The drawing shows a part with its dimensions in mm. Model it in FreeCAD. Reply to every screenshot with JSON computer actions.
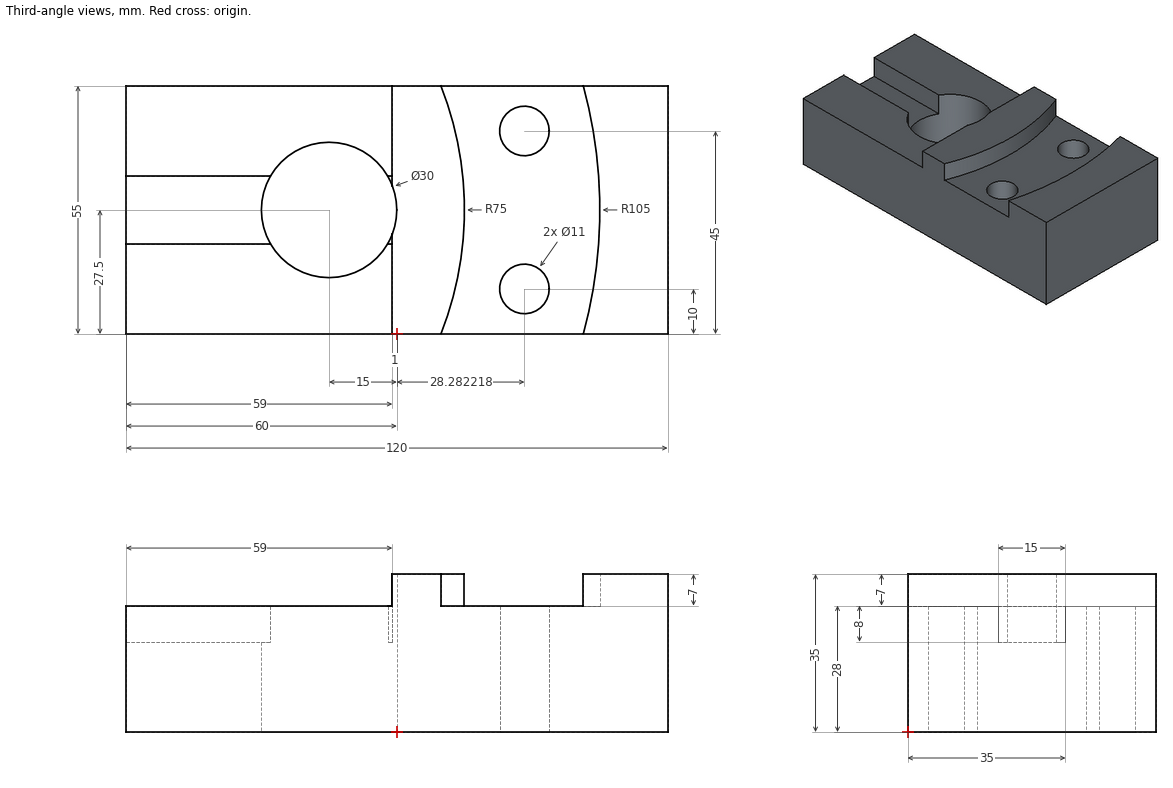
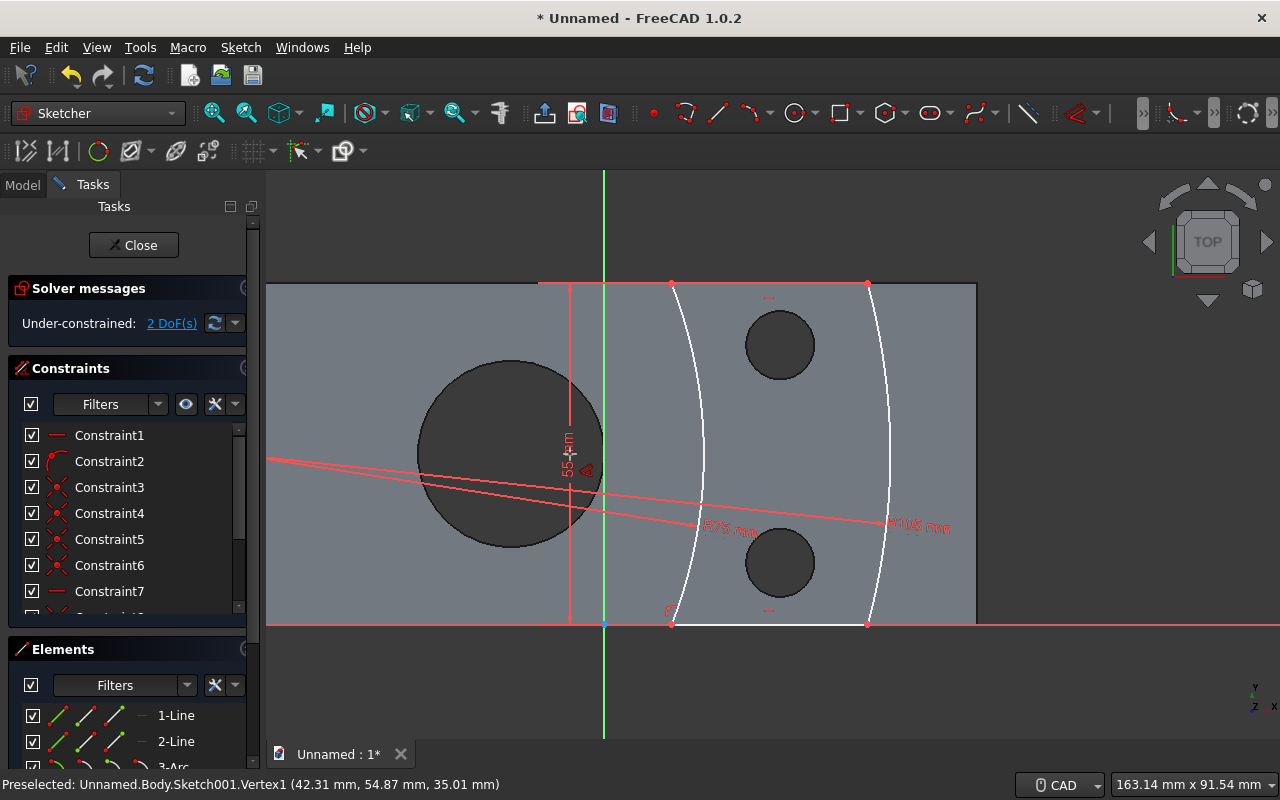
{"action": "scroll", "coordinate": [1115, 457], "scroll_direction": "down", "scroll_amount": 1}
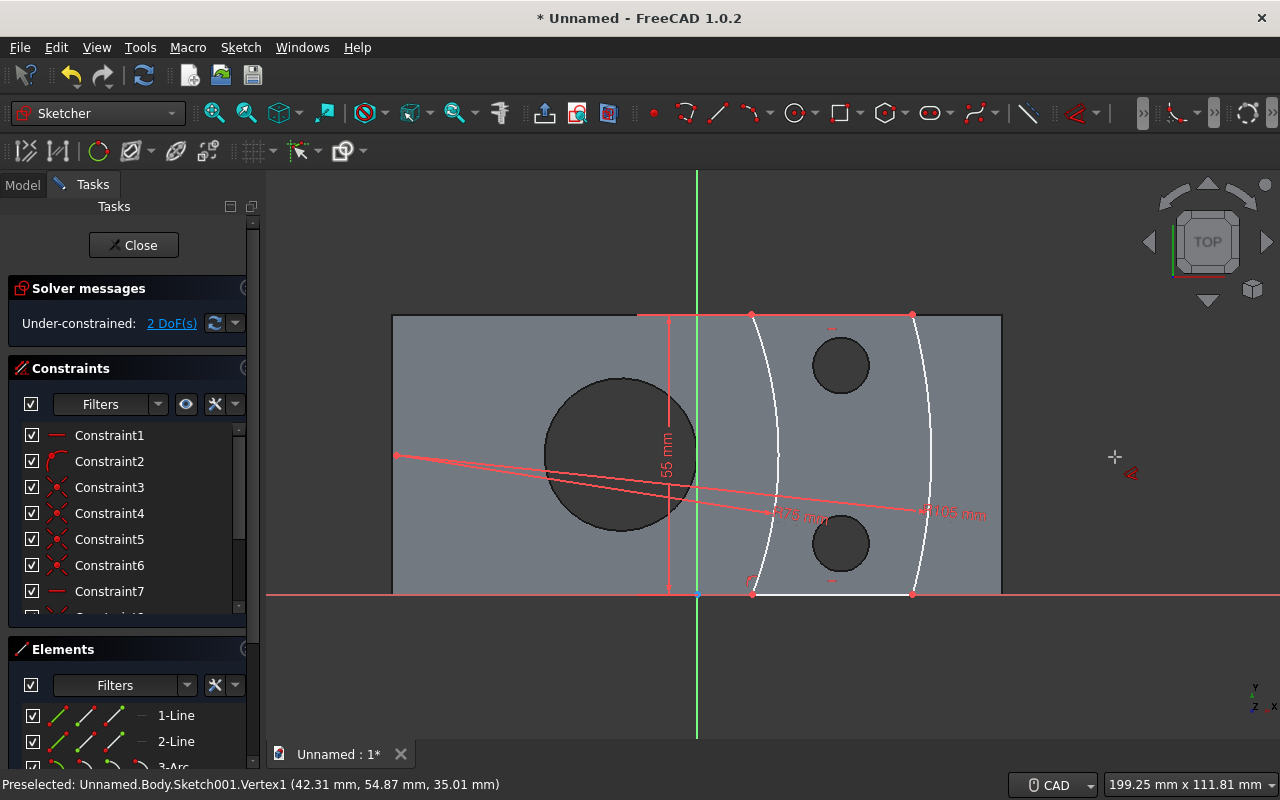
{"action": "left_click", "coordinate": [397, 455]}
{"action": "left_click", "coordinate": [547, 629]}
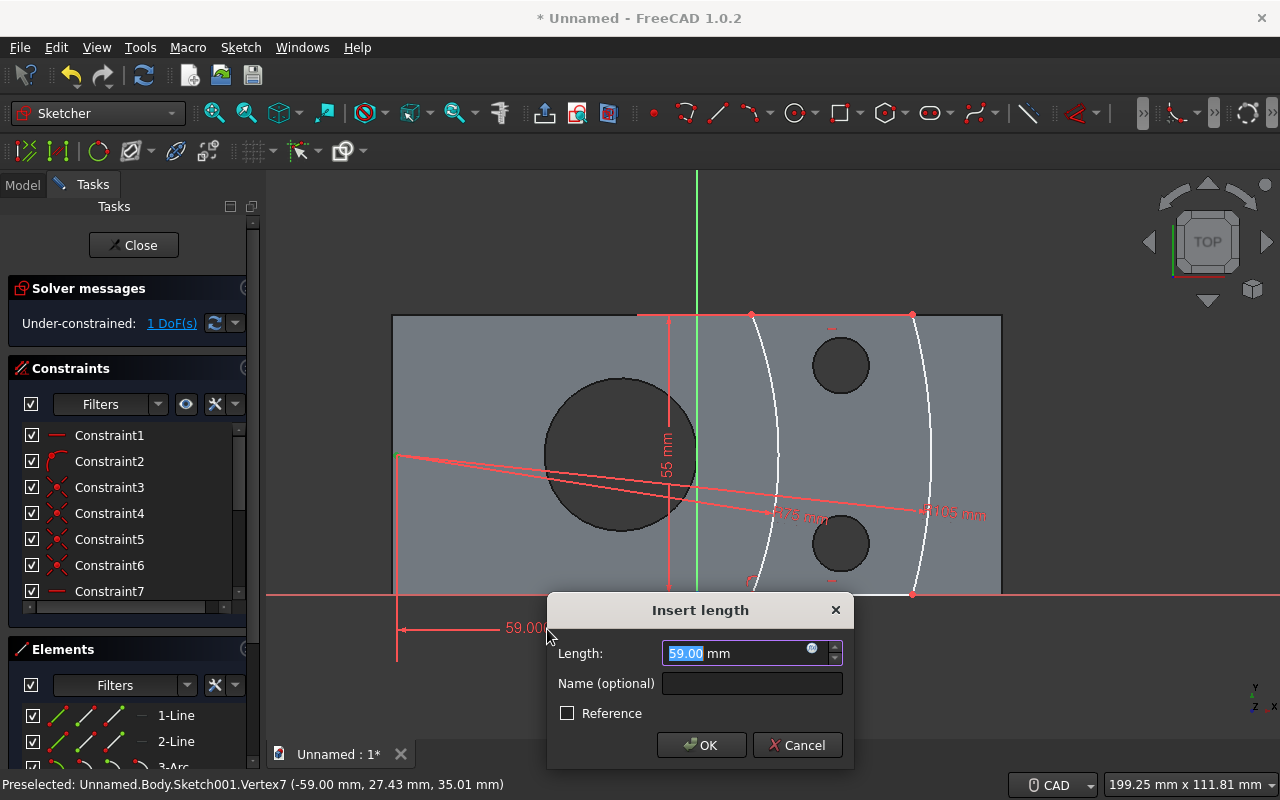
{"action": "type", "text": "60"}
{"action": "key", "text": "Return"}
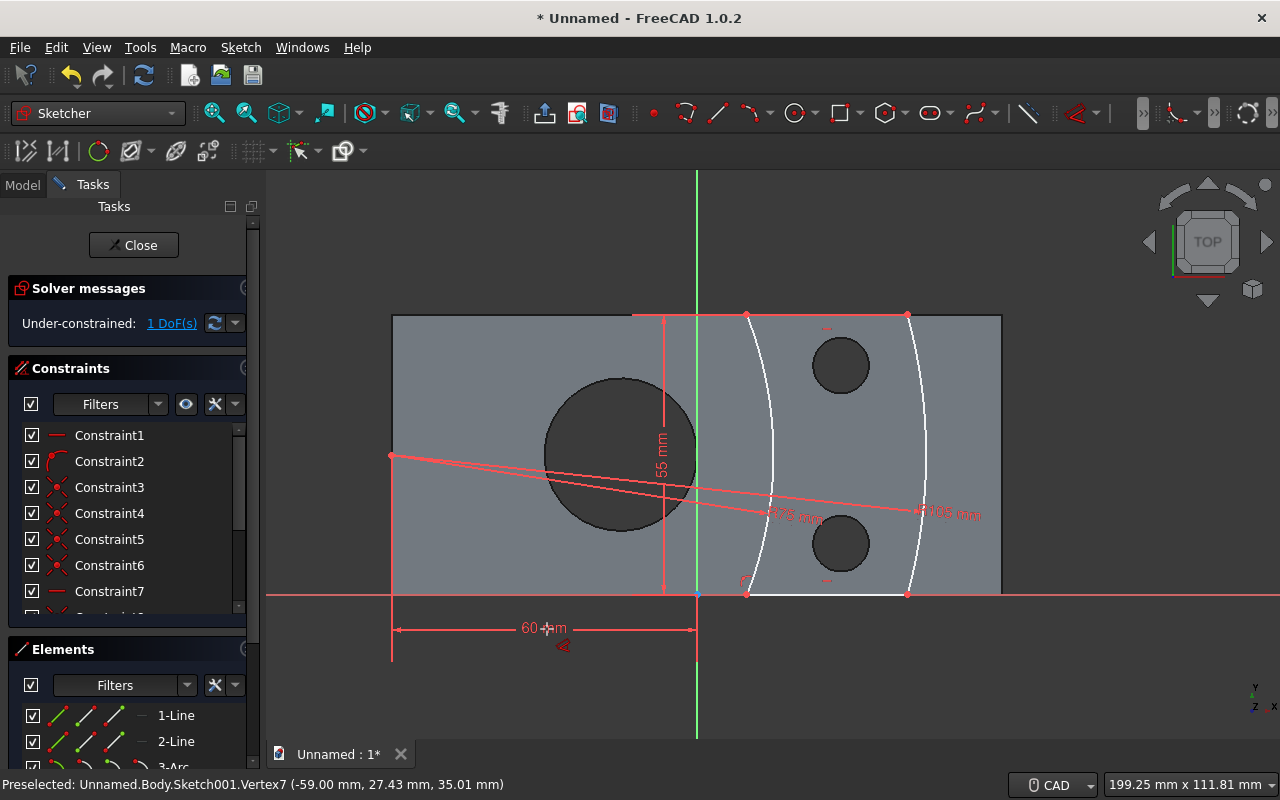
{"action": "left_click", "coordinate": [392, 455]}
{"action": "left_click", "coordinate": [358, 525]}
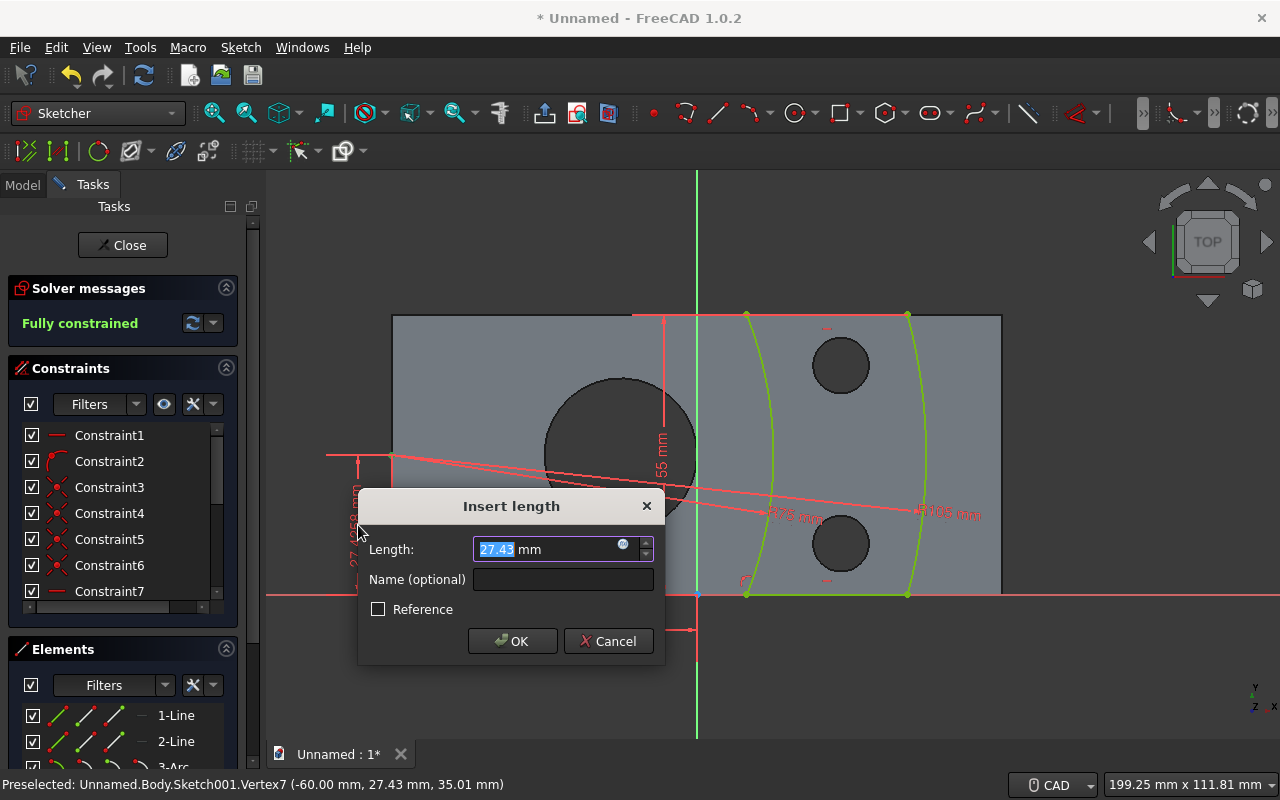
{"action": "type", "text": "27.5"}
{"action": "key", "text": "Return"}
{"action": "key", "text": "Escape"}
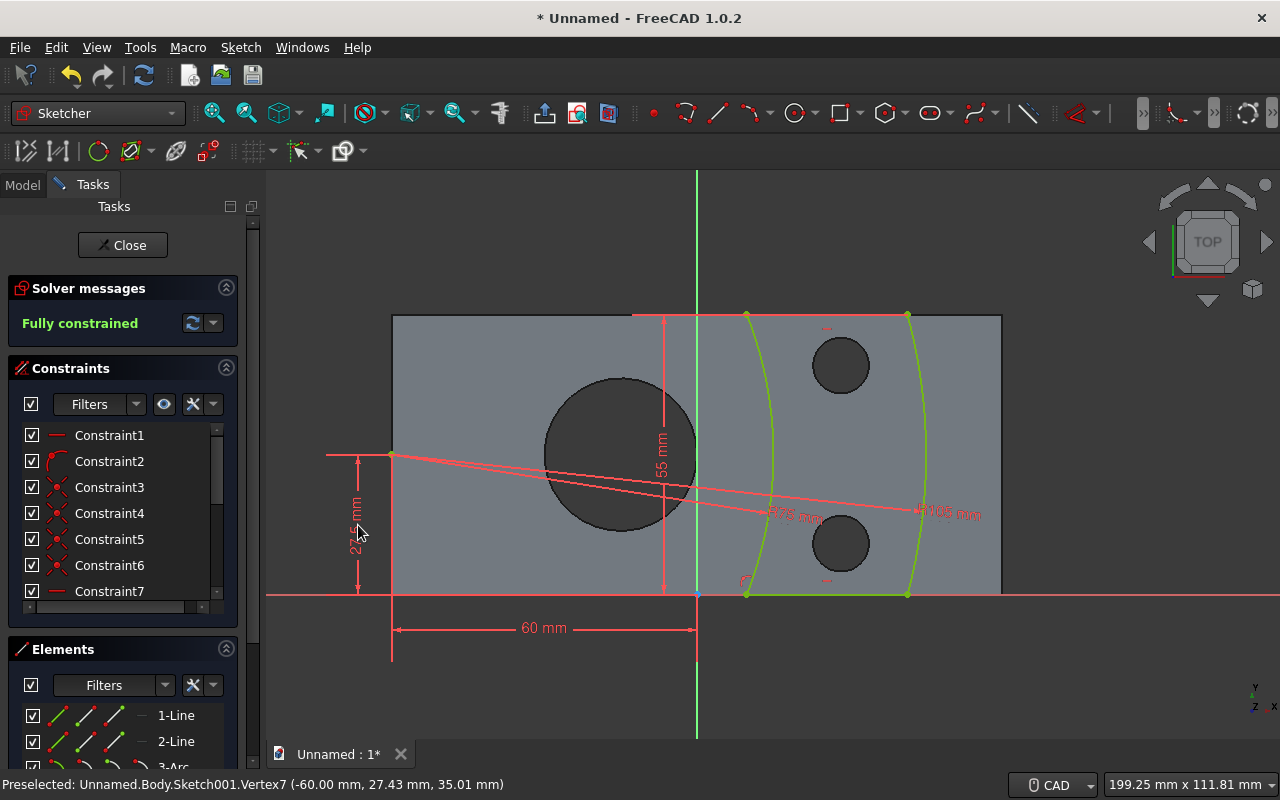
{"action": "left_click", "coordinate": [123, 245]}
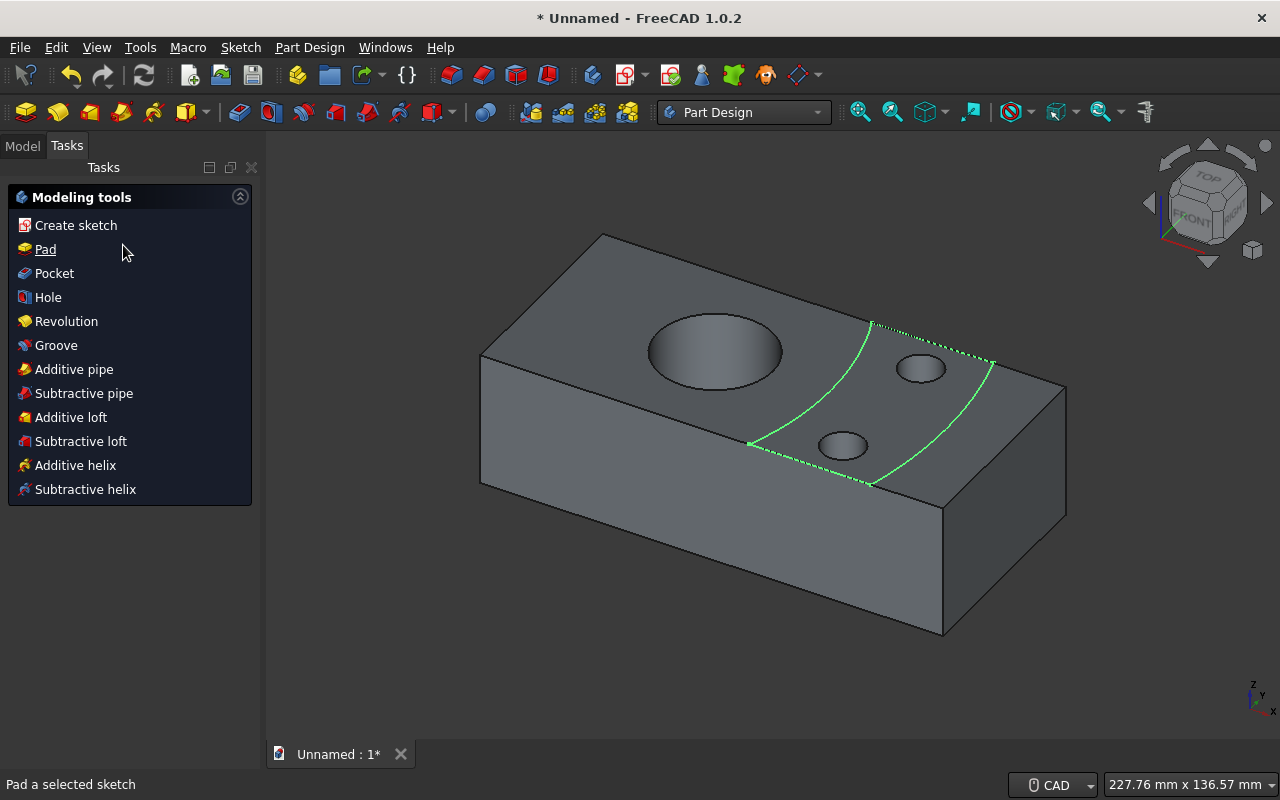
{"action": "left_click", "coordinate": [240, 112]}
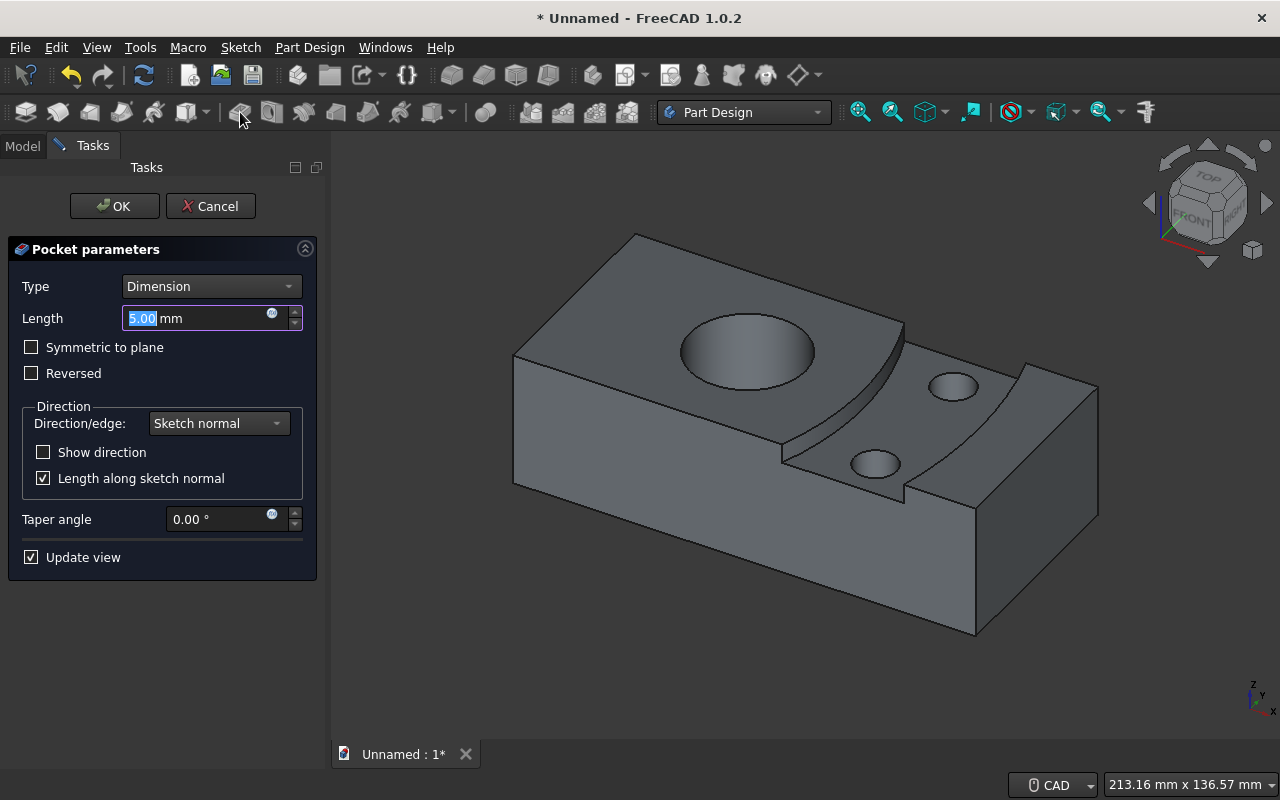
{"action": "type", "text": "7"}
{"action": "key", "text": "Tab"}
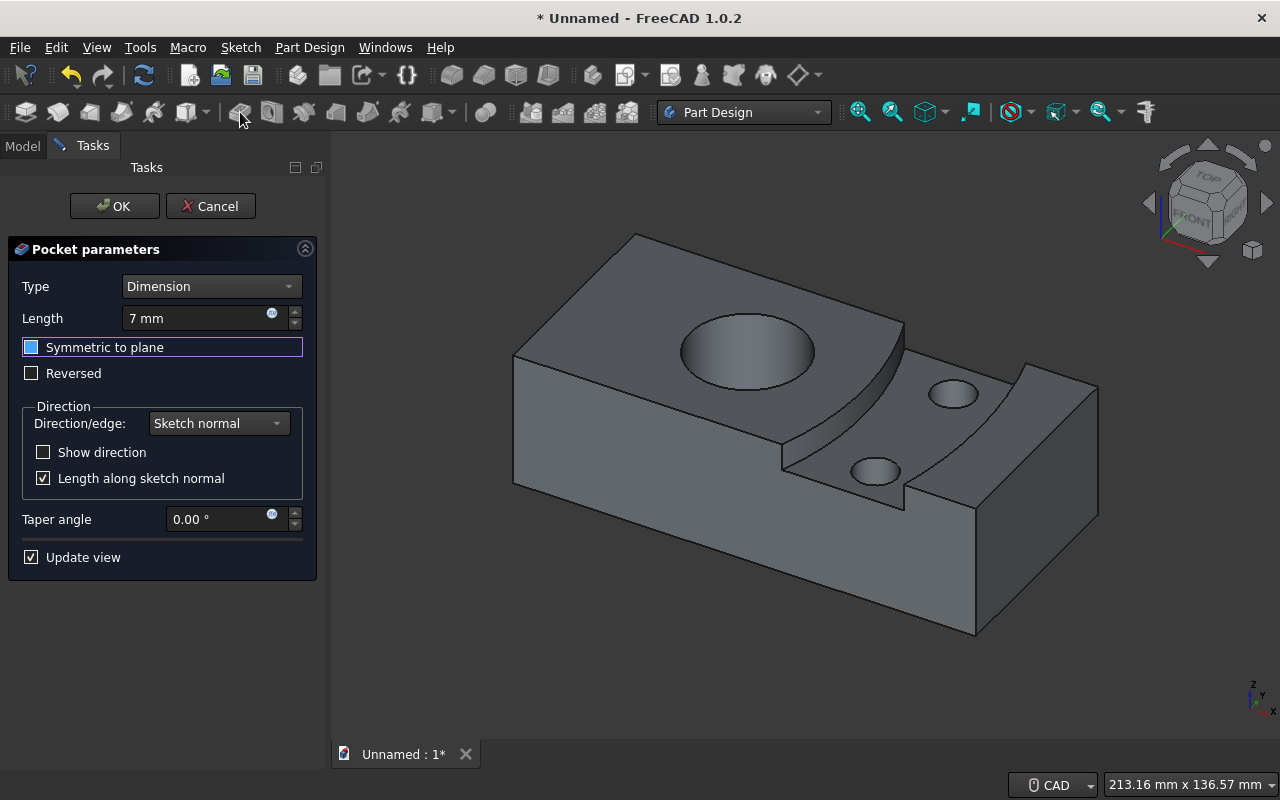
{"action": "left_click", "coordinate": [115, 206]}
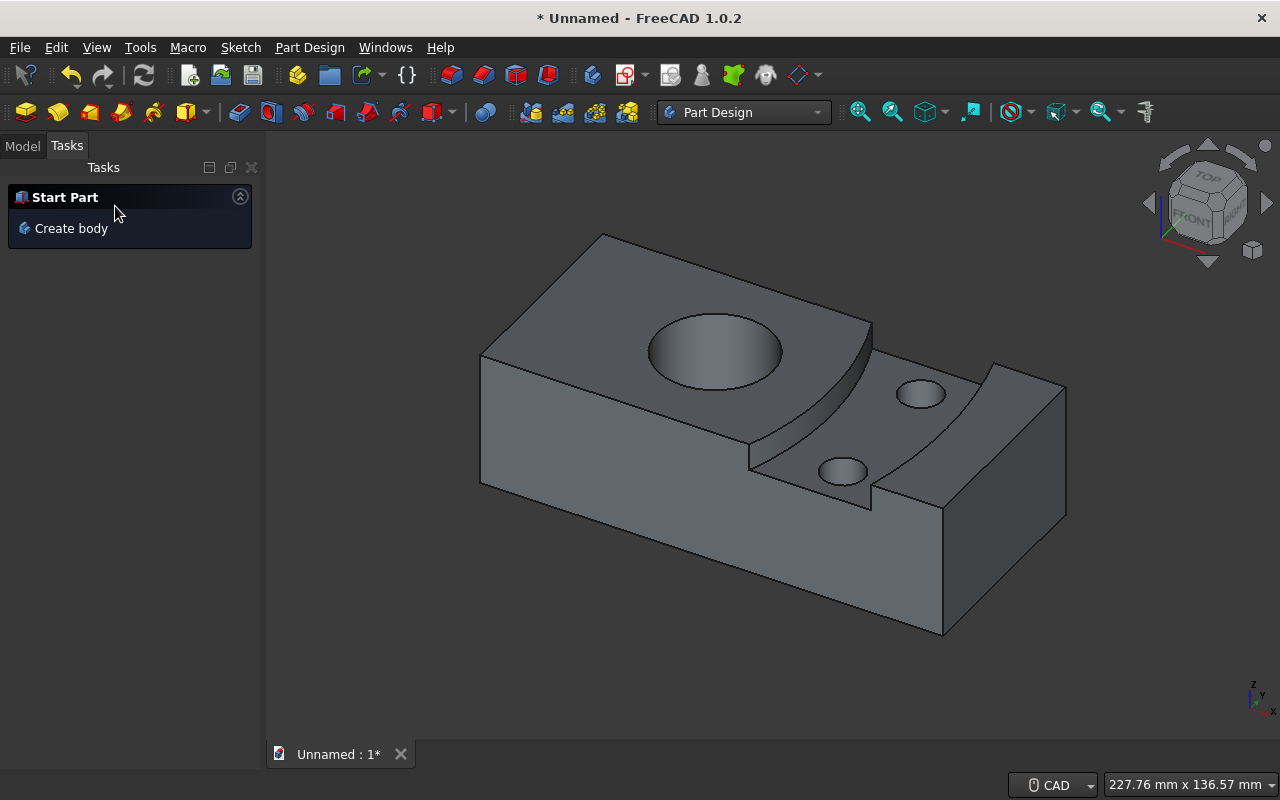
{"action": "left_click", "coordinate": [586, 331]}